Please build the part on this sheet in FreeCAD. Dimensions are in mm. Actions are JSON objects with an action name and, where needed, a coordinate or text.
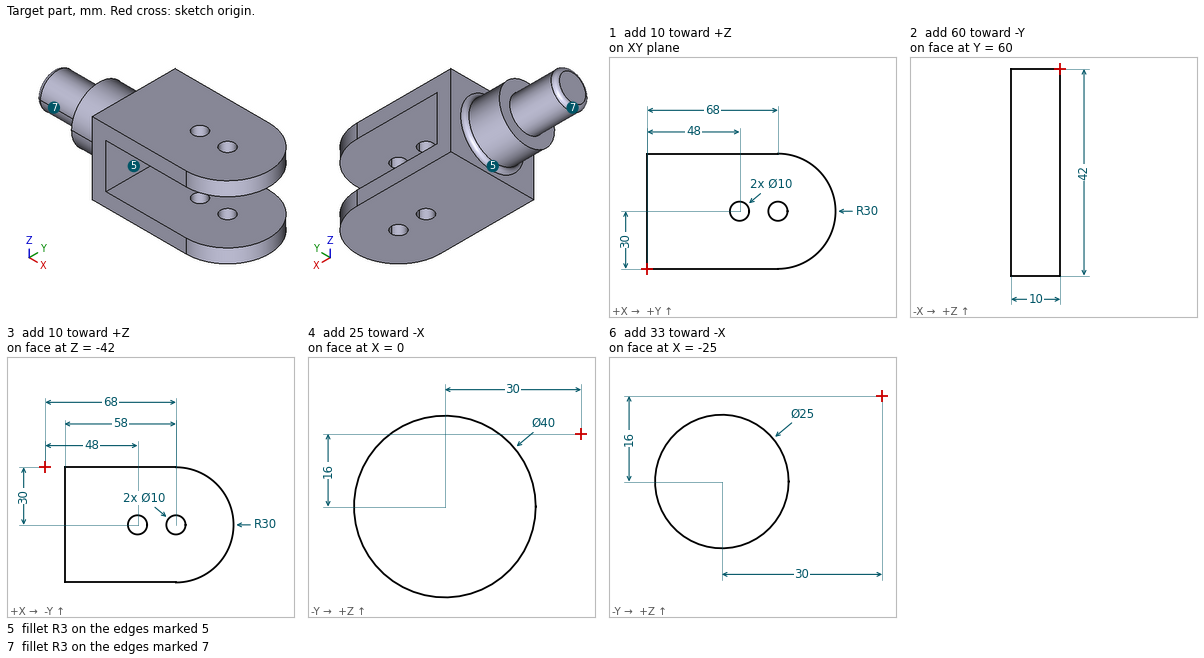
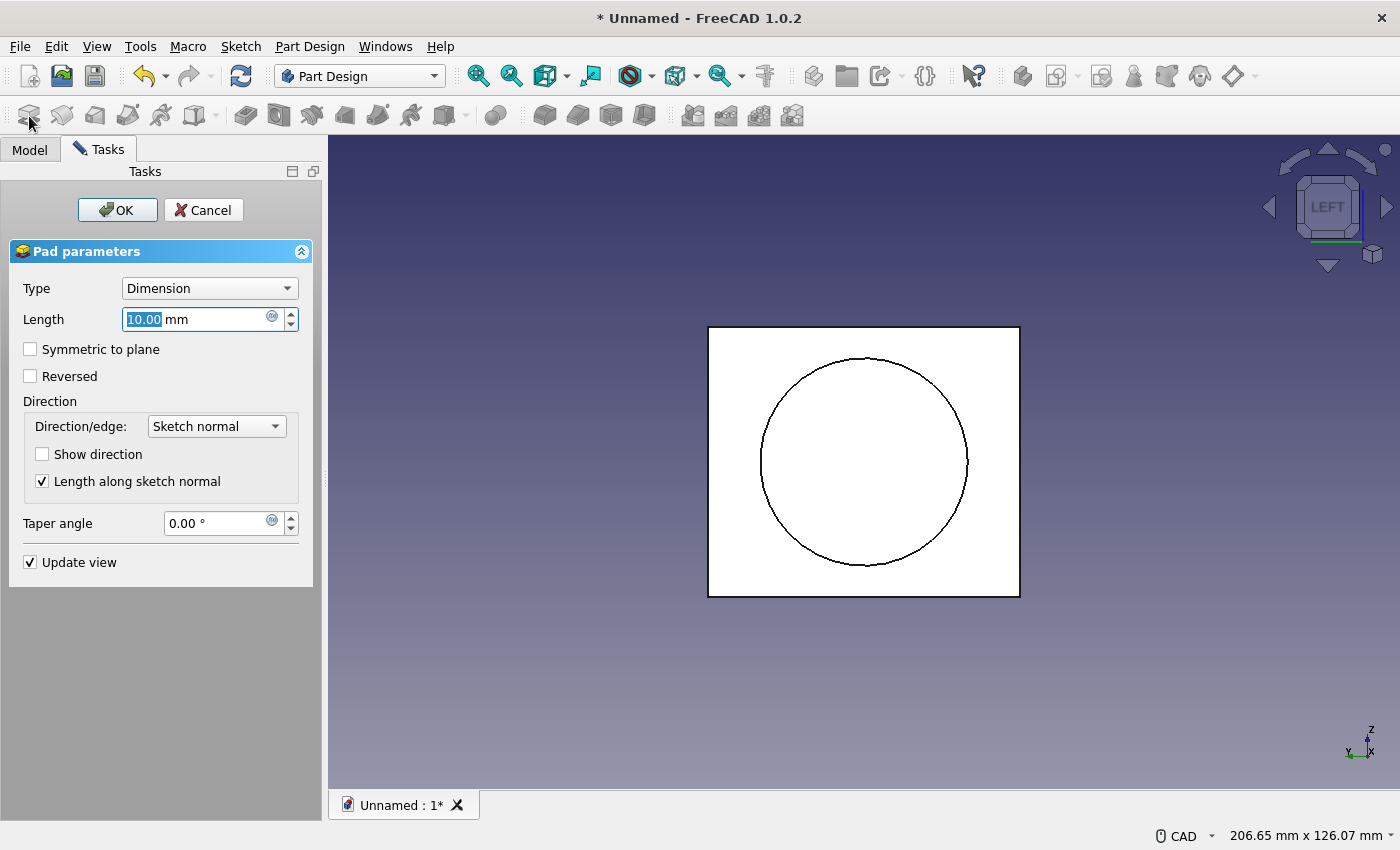
{"action": "type", "text": "25"}
{"action": "key", "text": "Tab"}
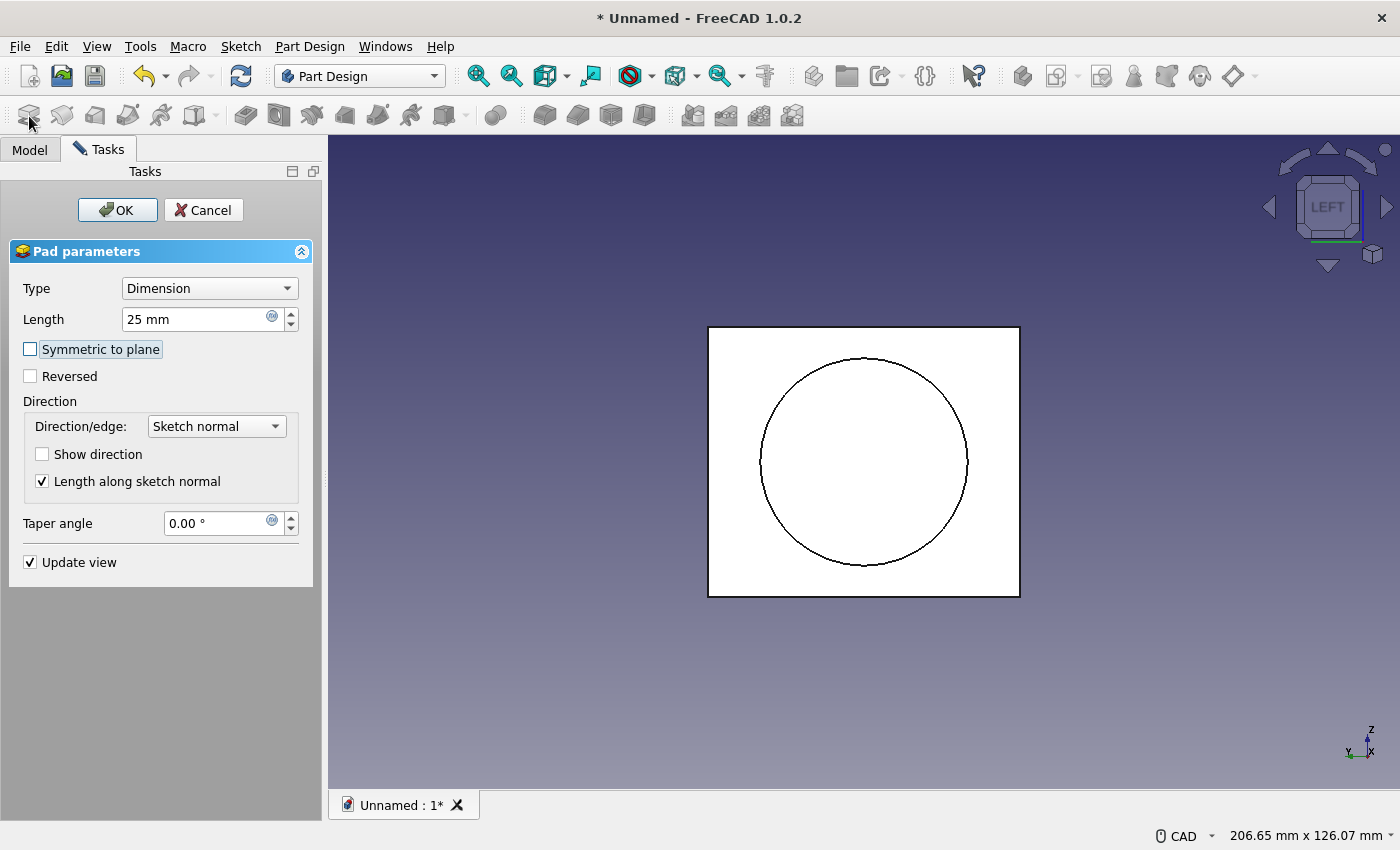
{"action": "left_click", "coordinate": [118, 210]}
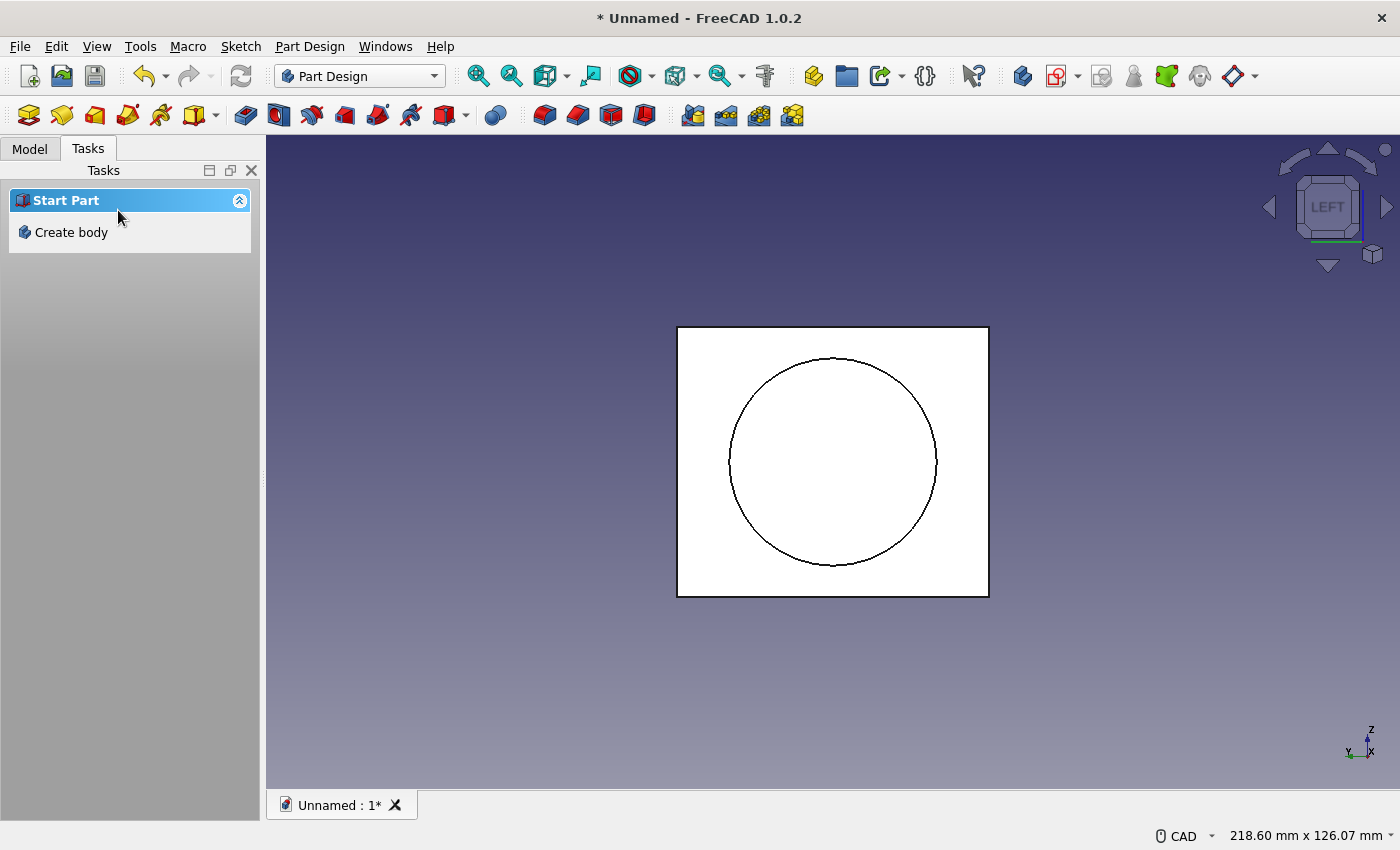
{"action": "left_click", "coordinate": [479, 76]}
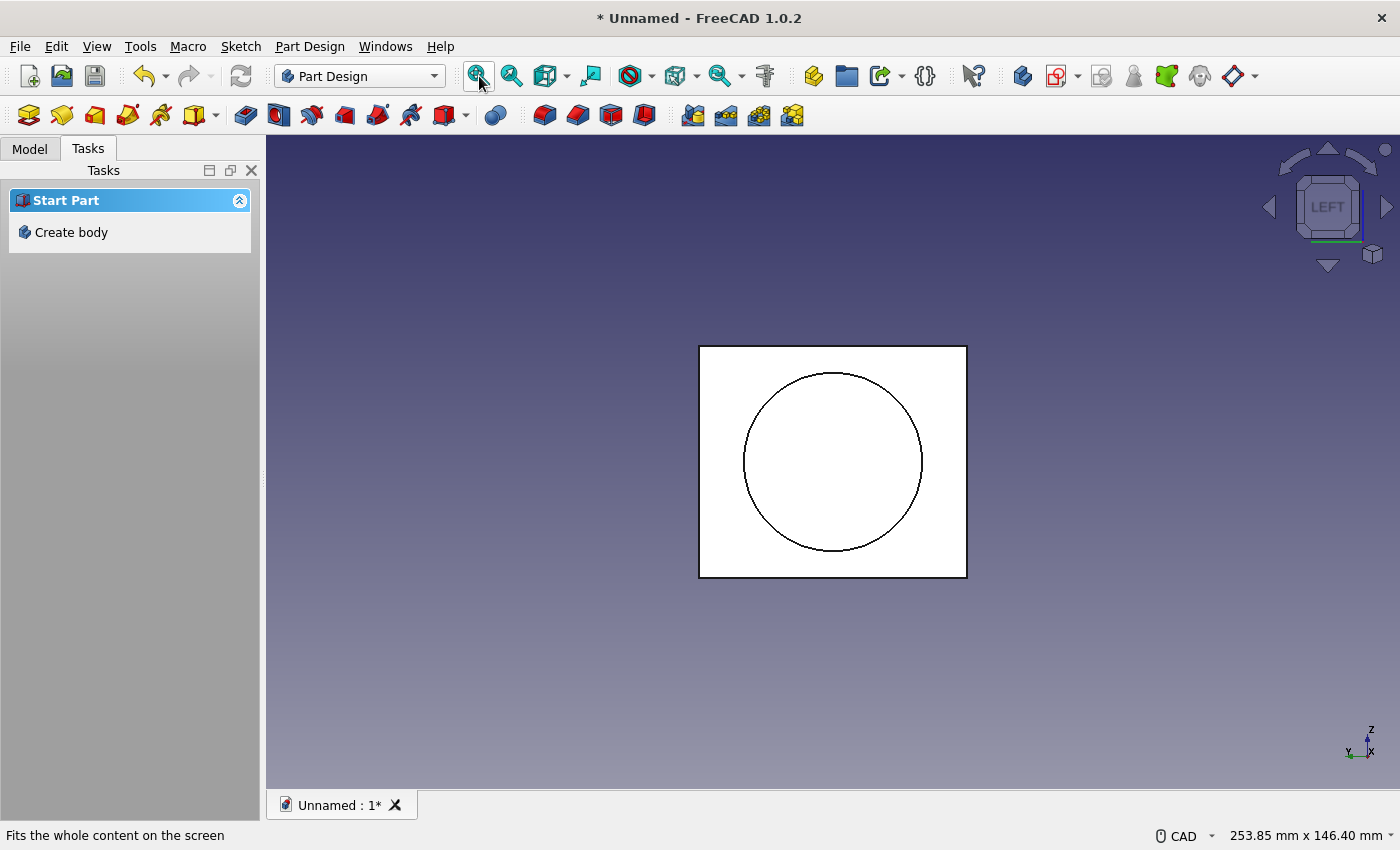
{"action": "key", "text": "0"}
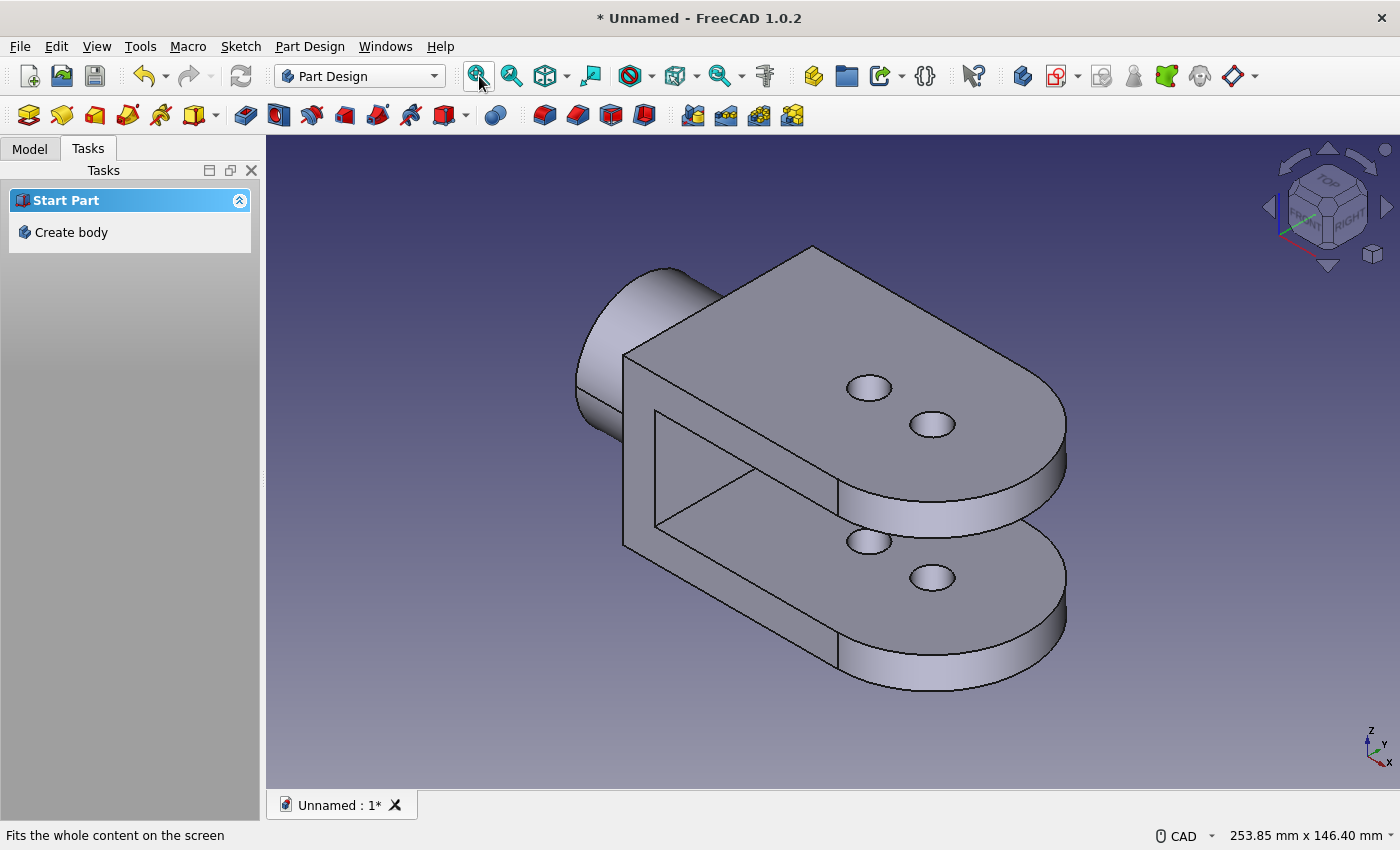
{"action": "key", "text": "2"}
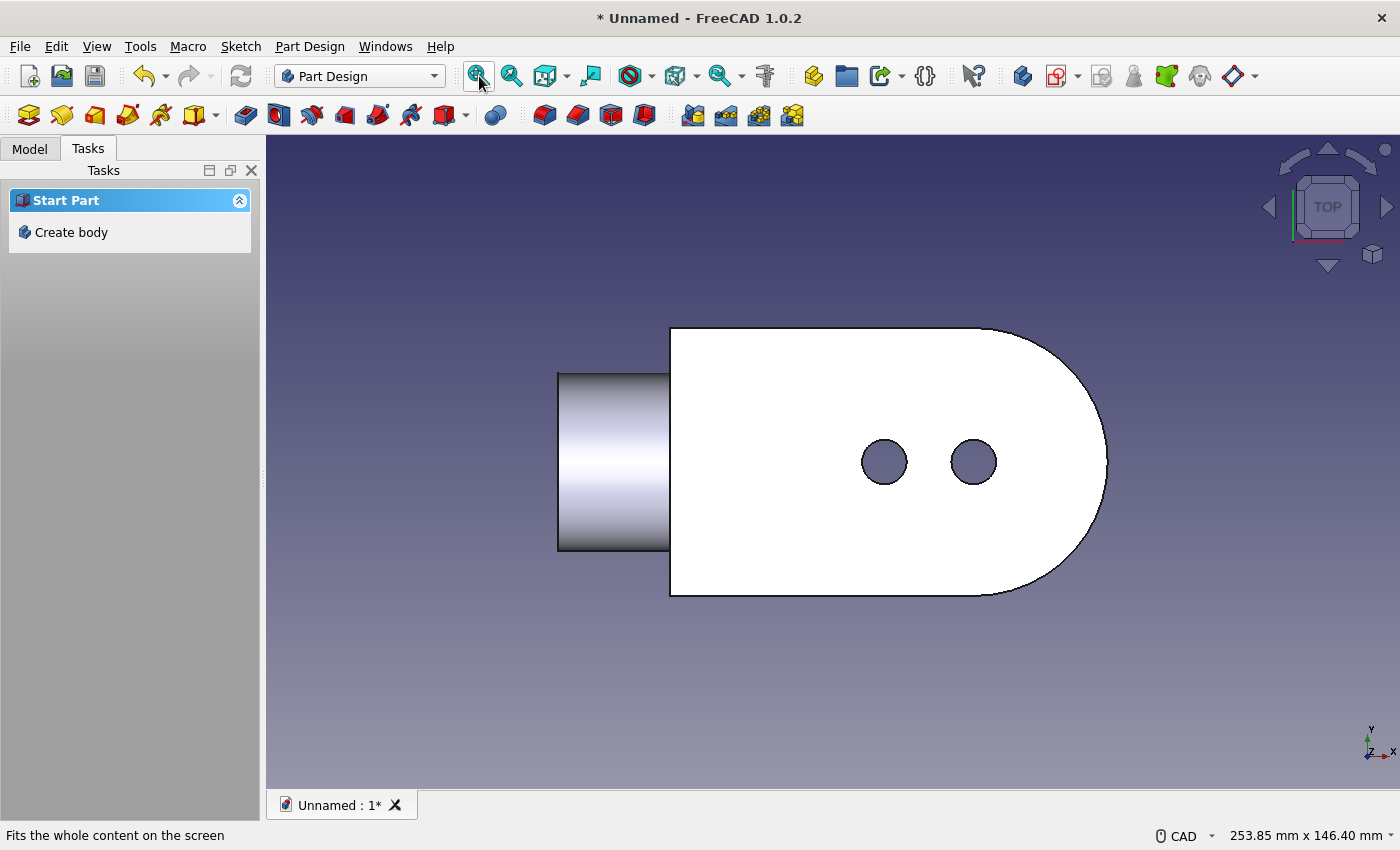
{"action": "key", "text": "1"}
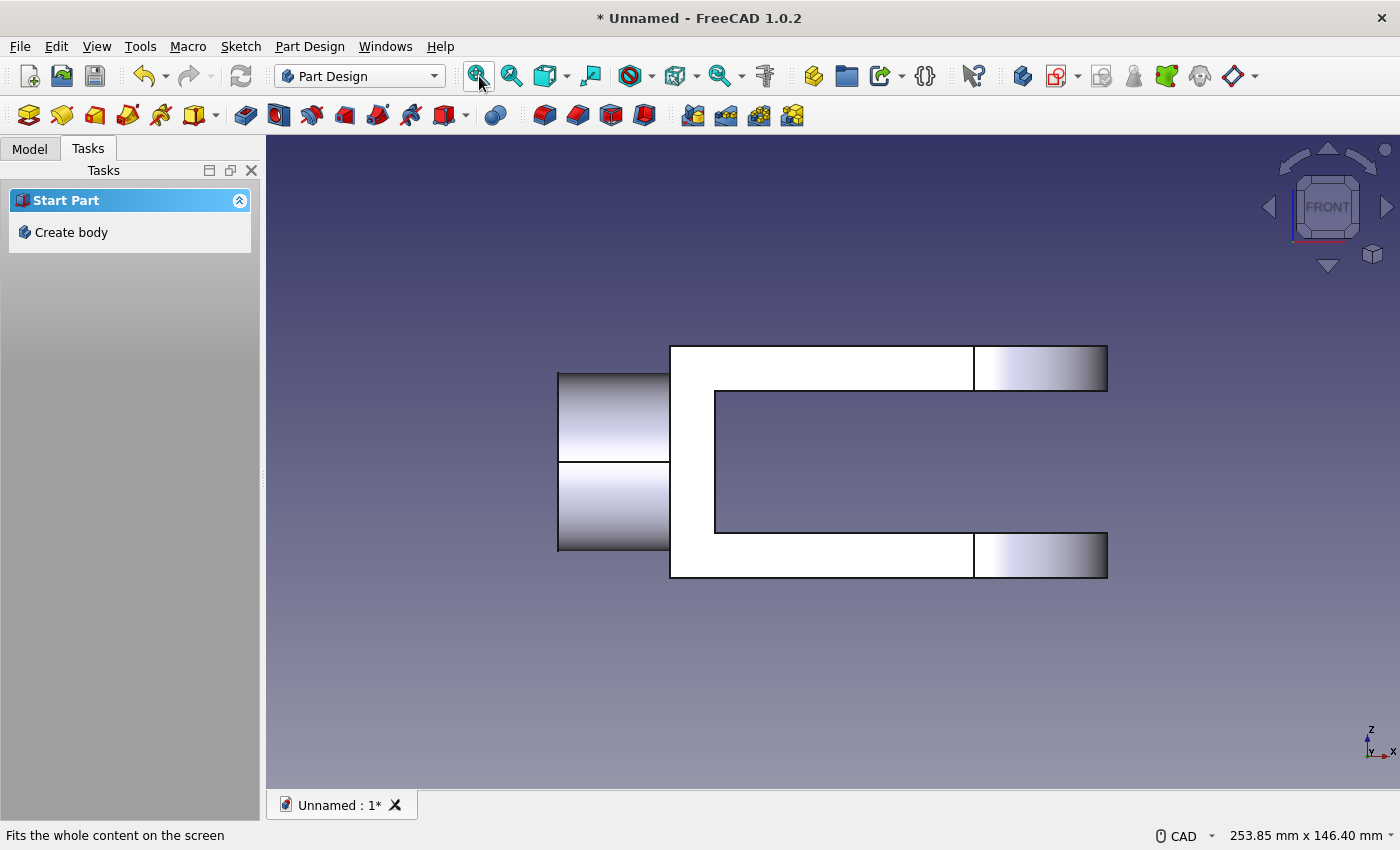
{"action": "key", "text": "3"}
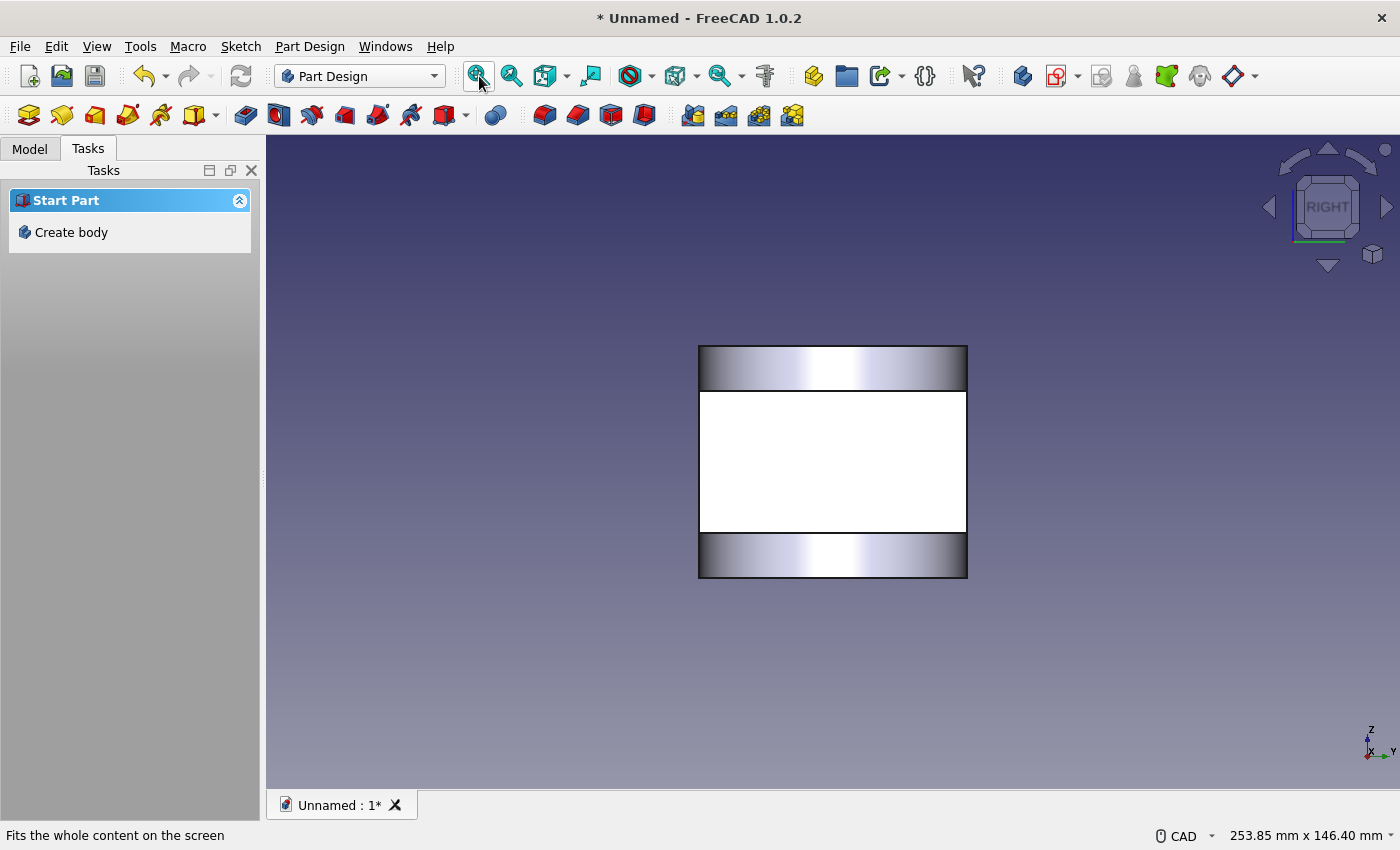
{"action": "key", "text": "v f"}